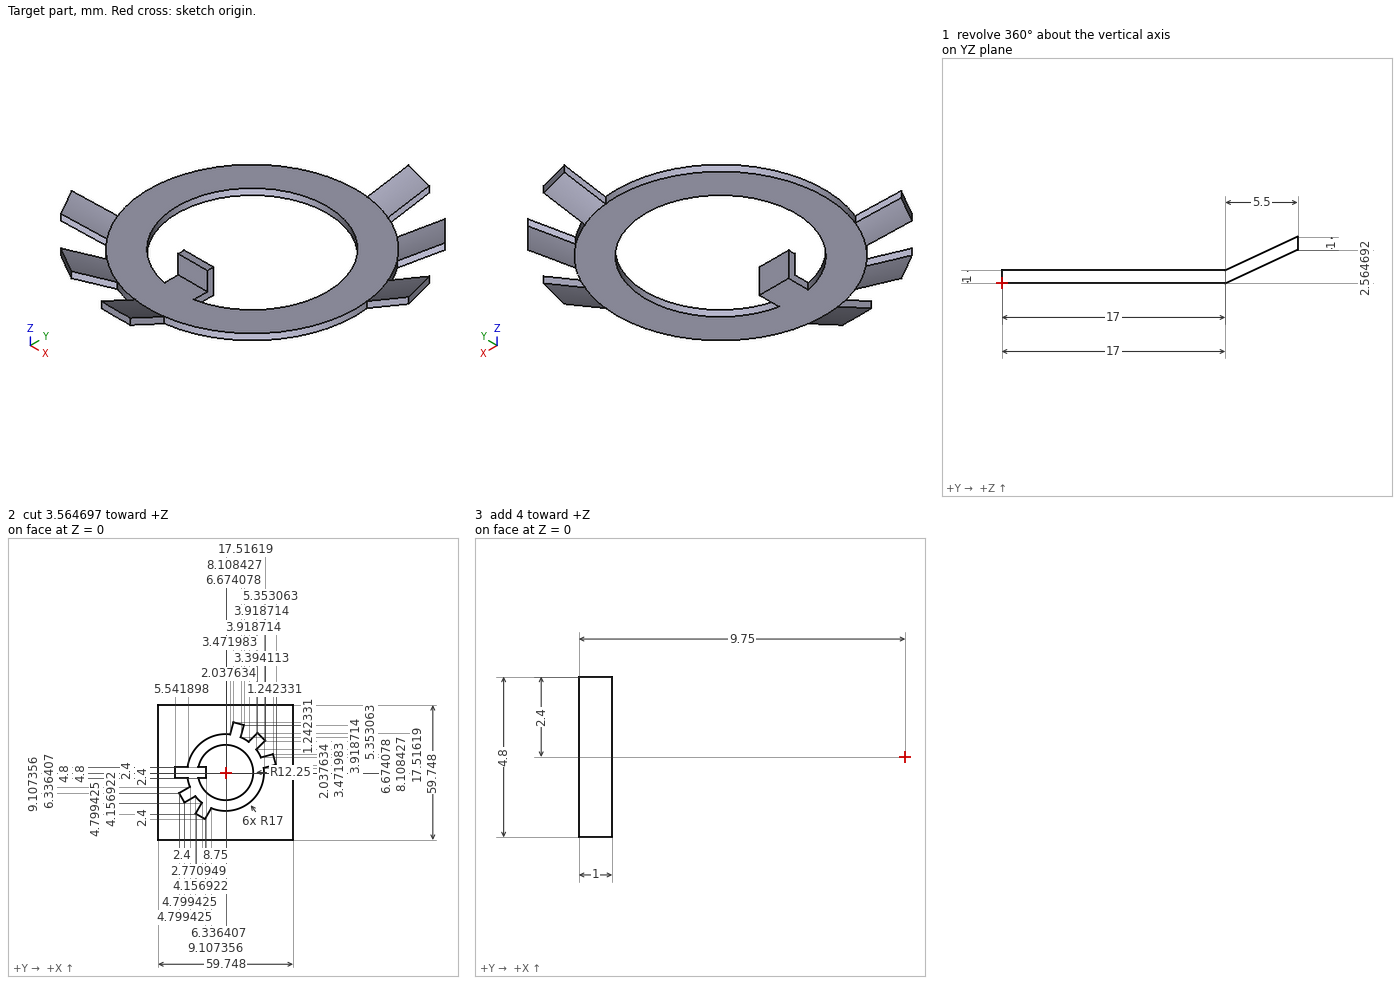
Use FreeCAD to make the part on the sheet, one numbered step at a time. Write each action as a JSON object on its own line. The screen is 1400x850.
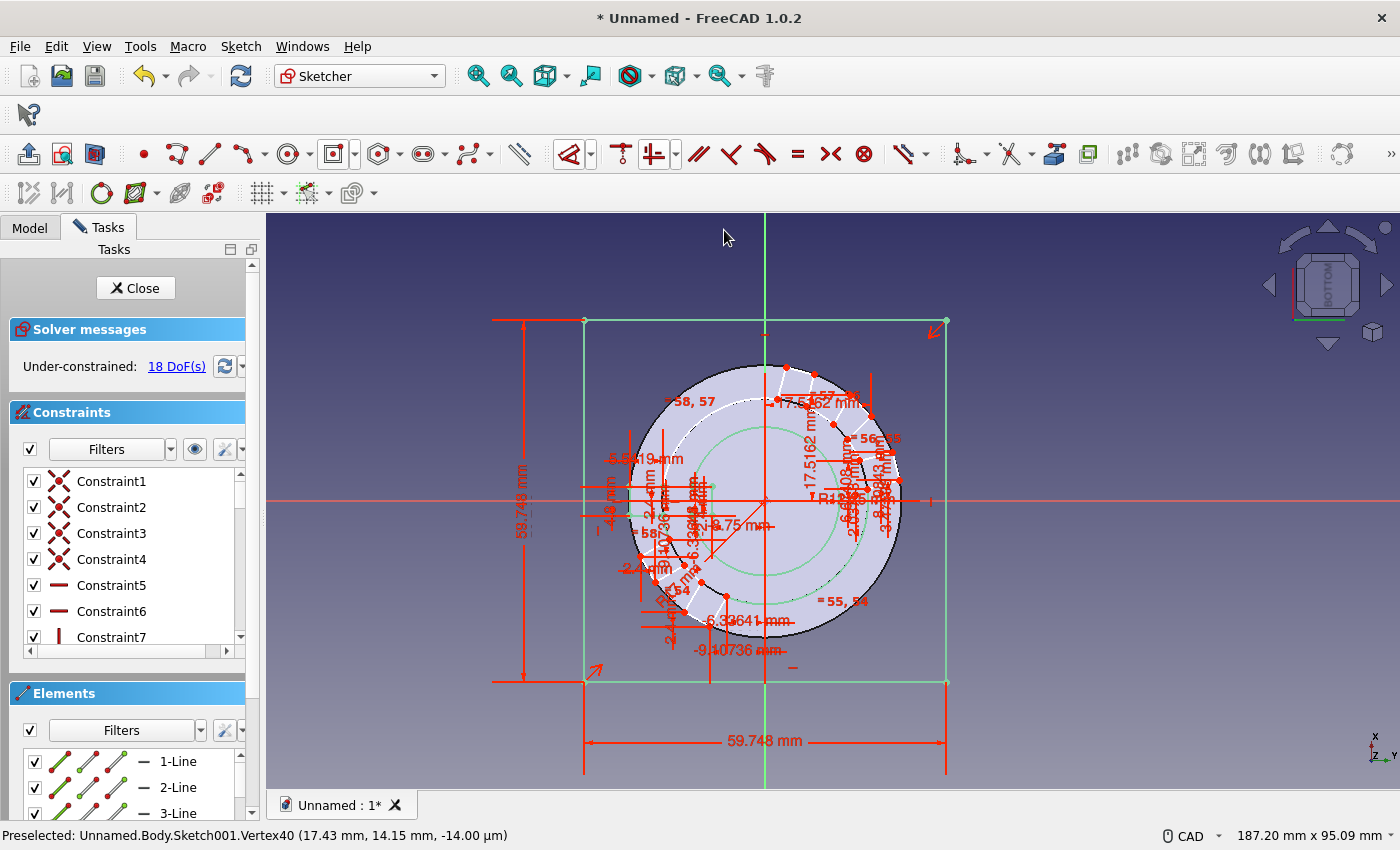
{"action": "left_click", "coordinate": [806, 407]}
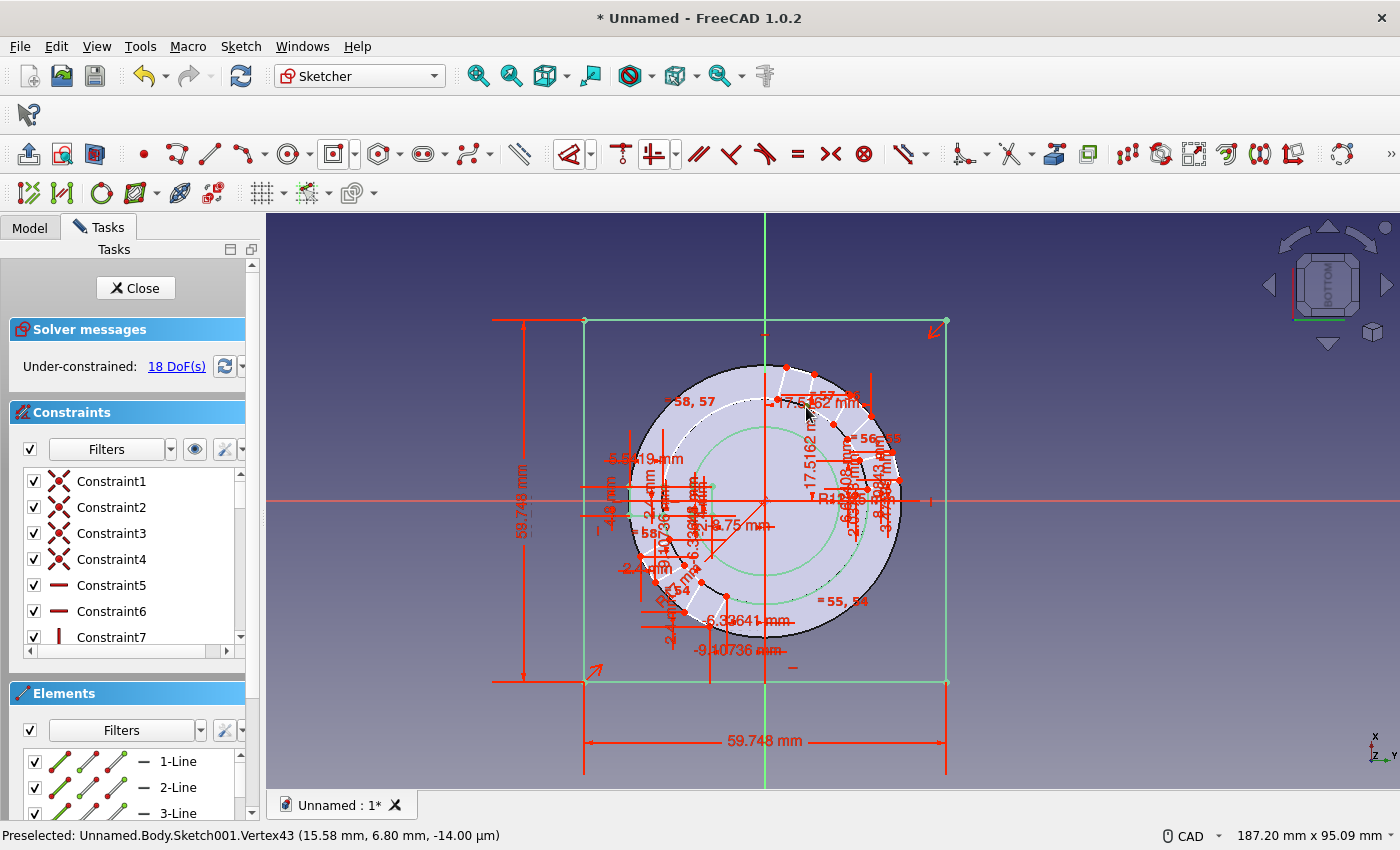
{"action": "left_click", "coordinate": [590, 154]}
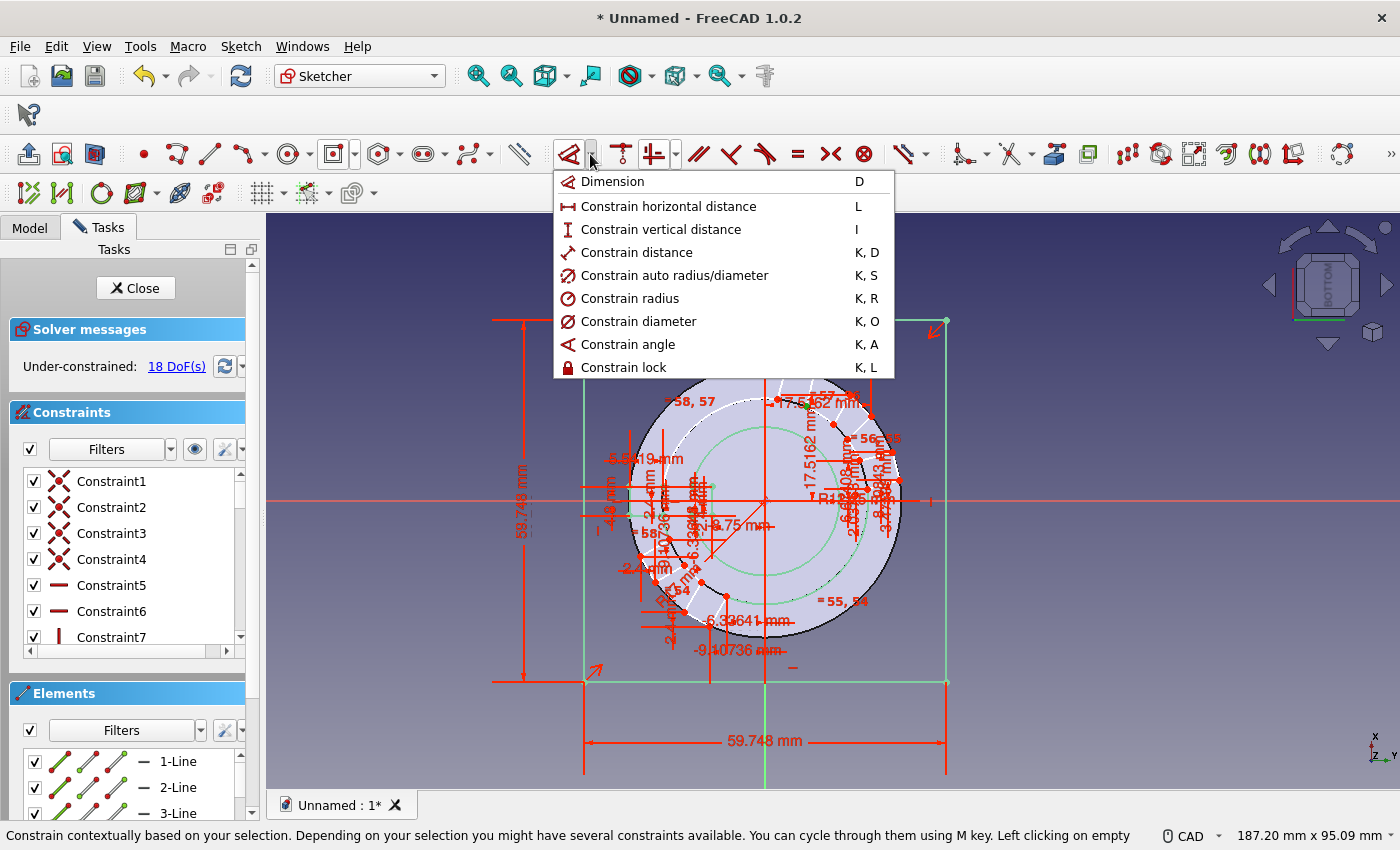
{"action": "left_click", "coordinate": [724, 206]}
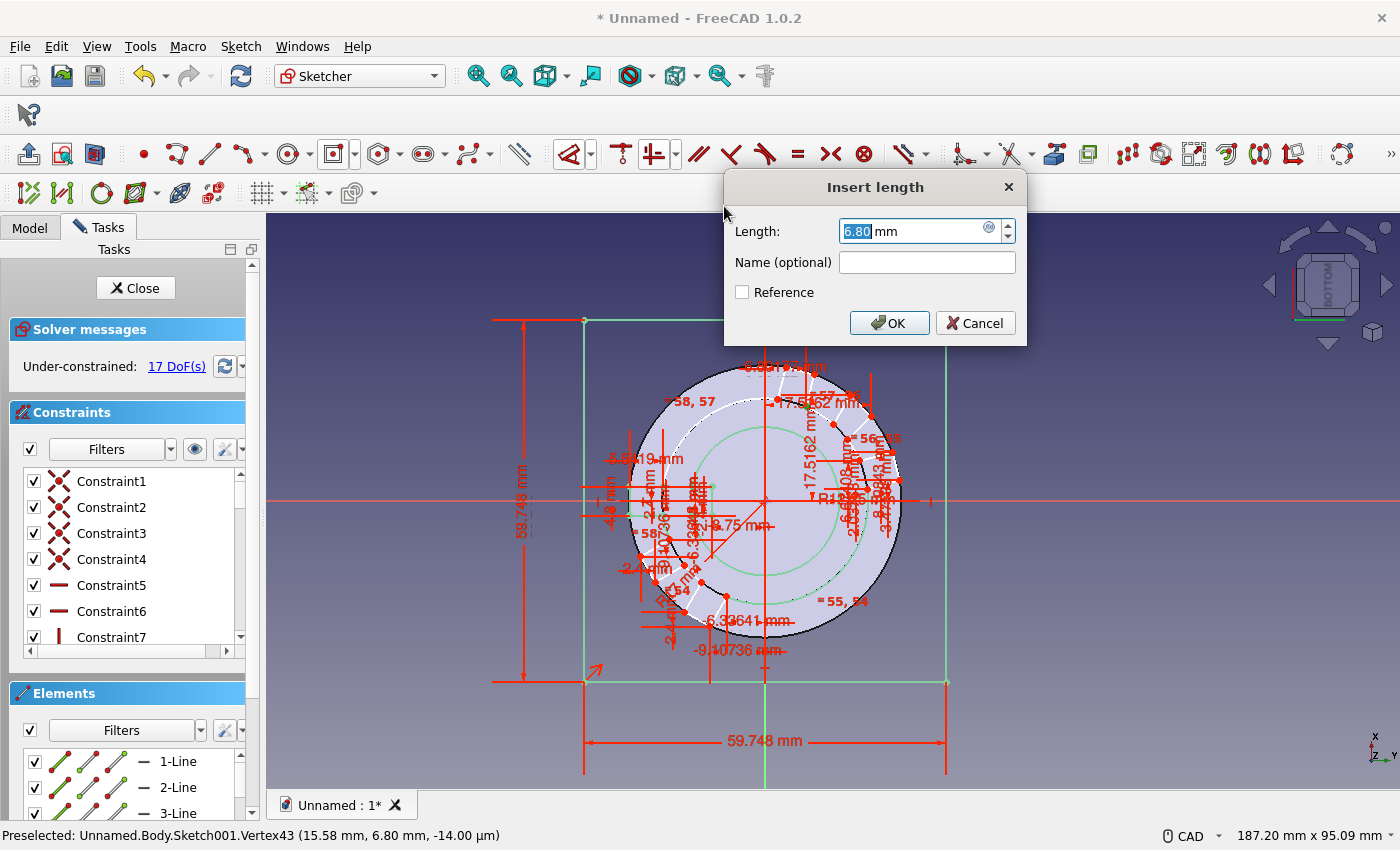
{"action": "type", "text": "6.674078"}
{"action": "key", "text": "Return"}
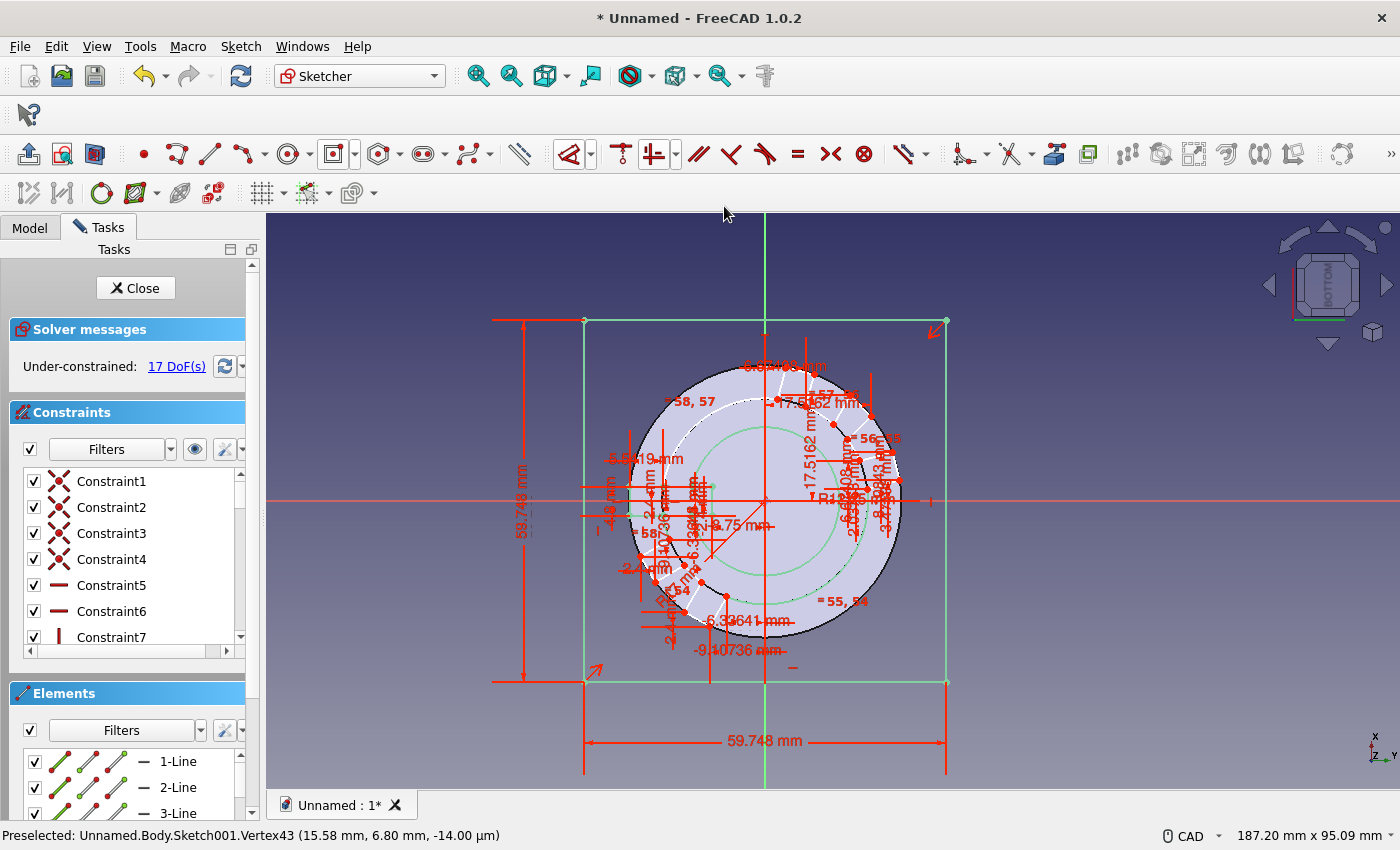
{"action": "left_click", "coordinate": [814, 375]}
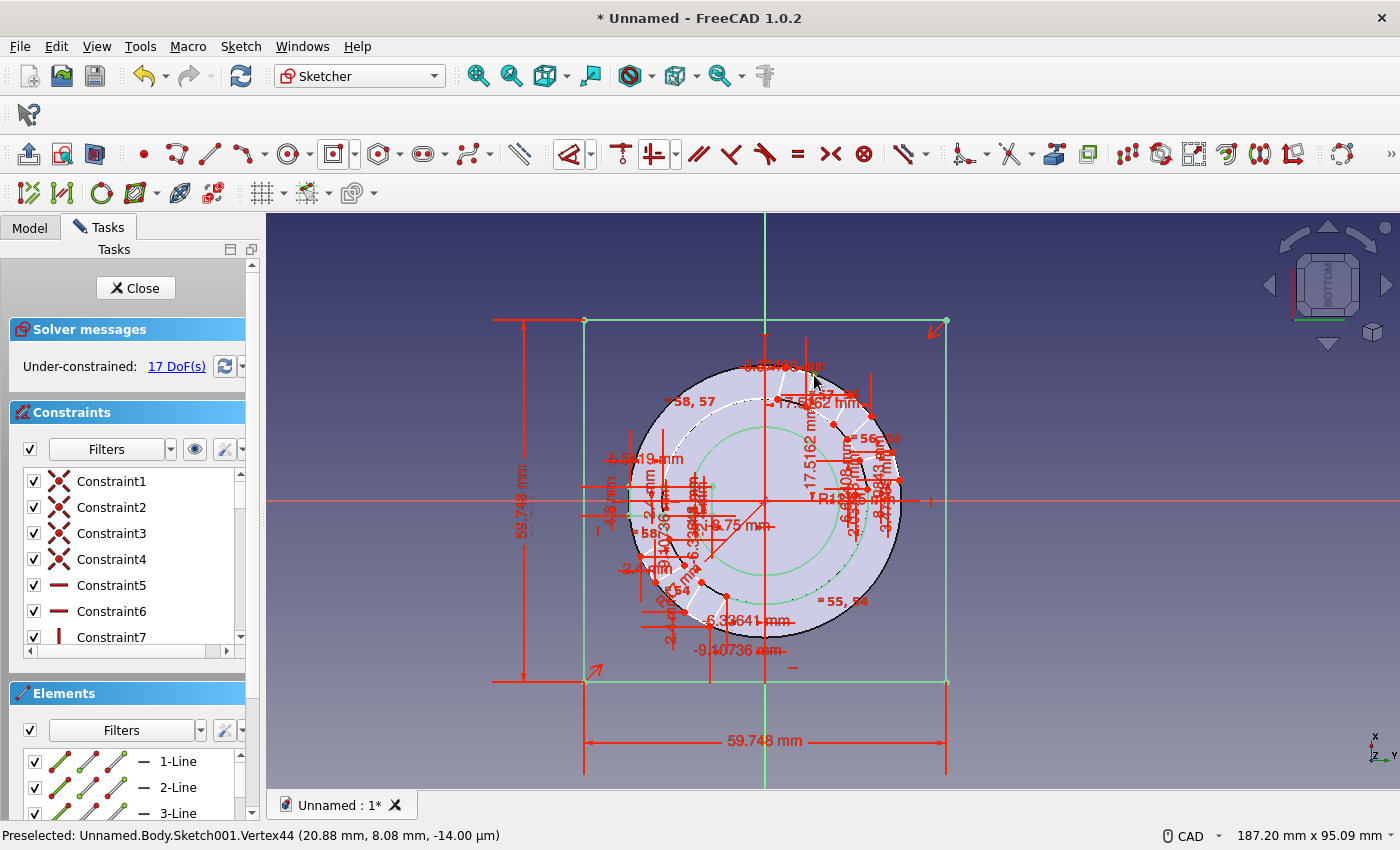
{"action": "key", "text": "l"}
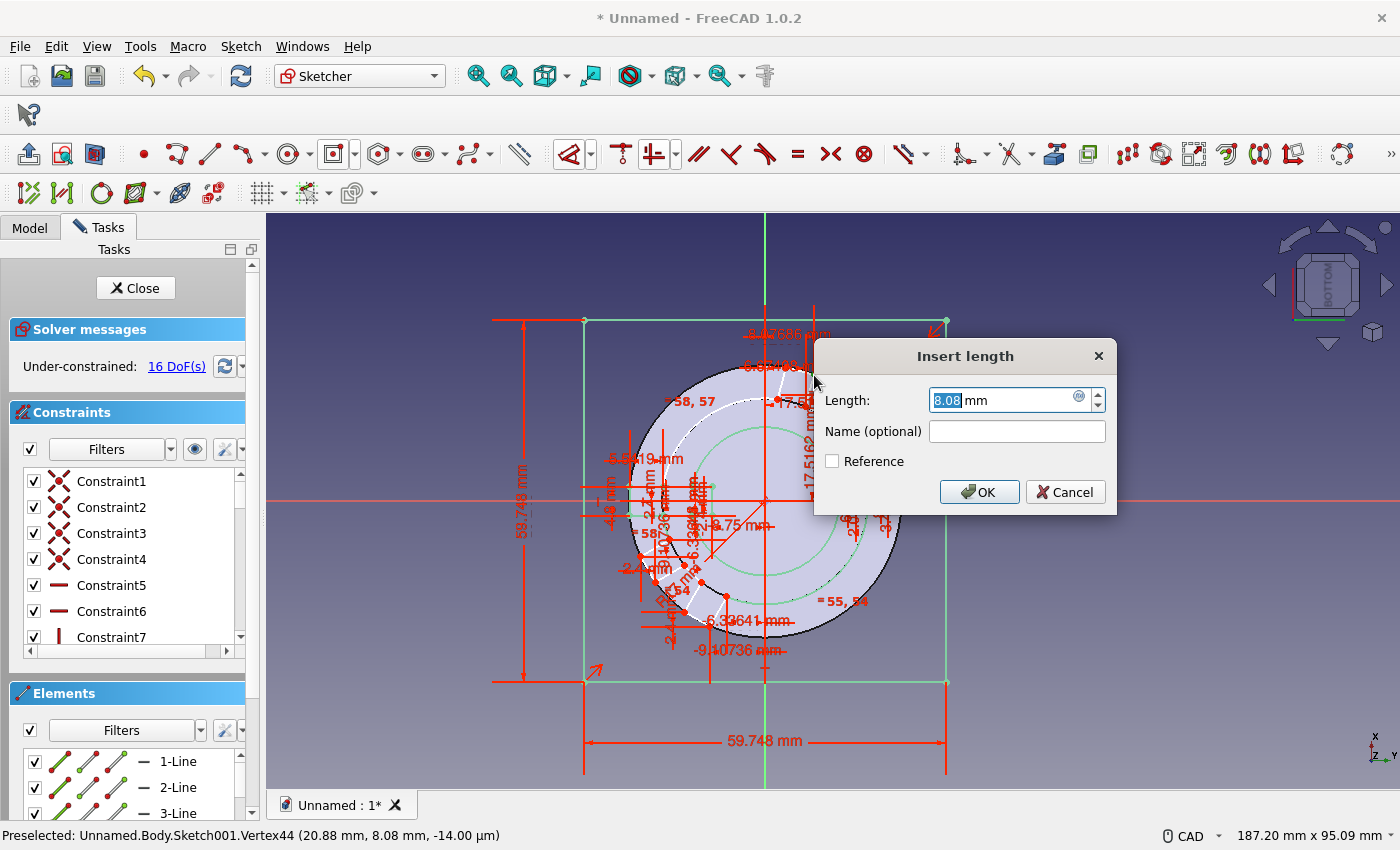
{"action": "type", "text": "8.108427"}
{"action": "key", "text": "Return"}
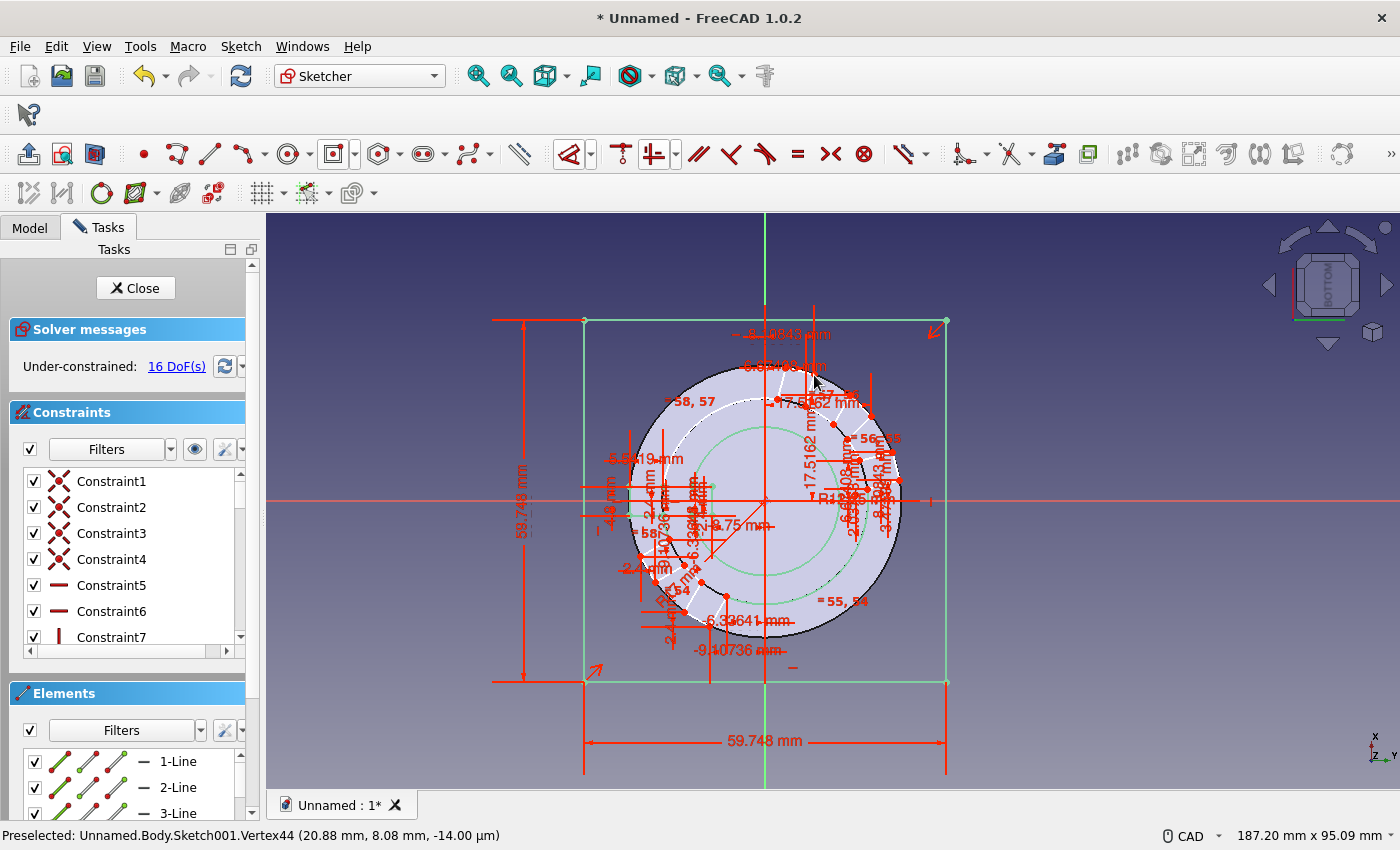
{"action": "scroll", "coordinate": [786, 367], "scroll_direction": "up", "scroll_amount": 4}